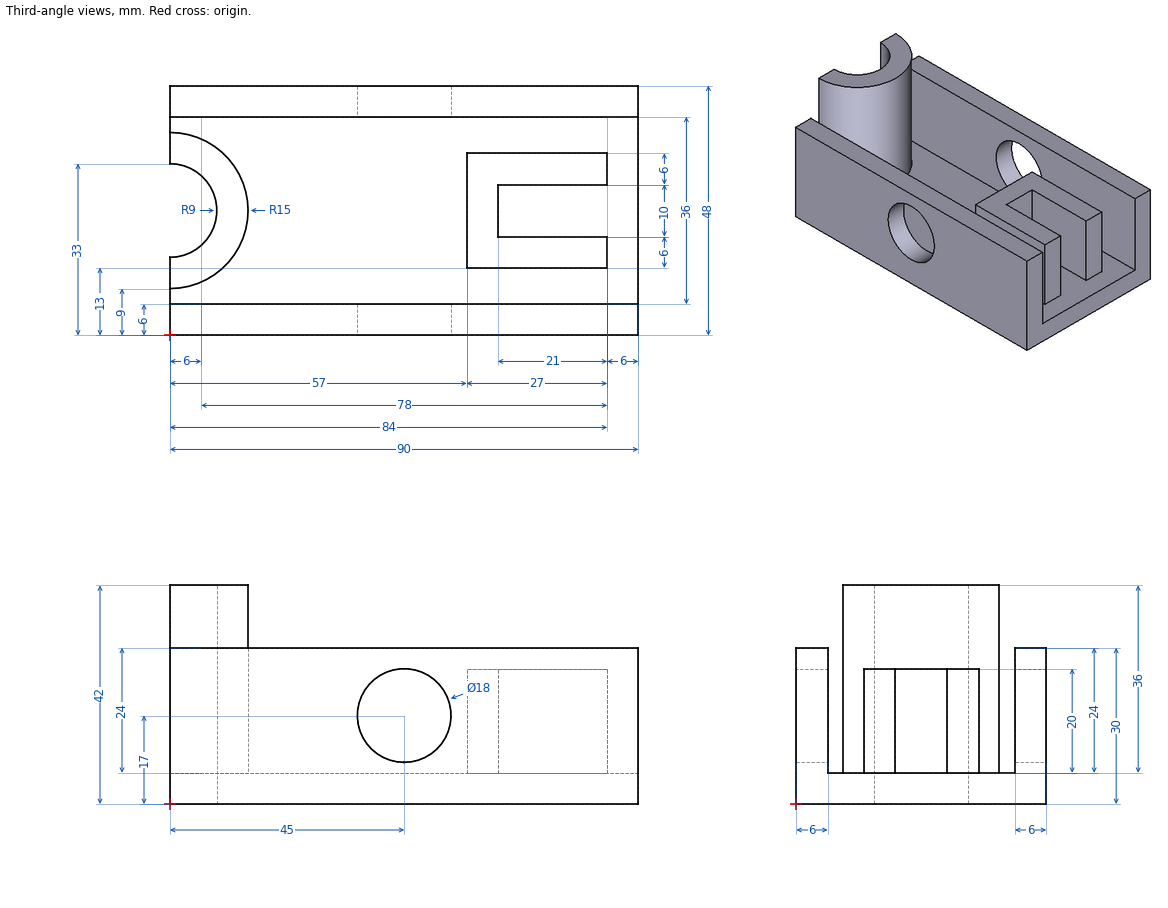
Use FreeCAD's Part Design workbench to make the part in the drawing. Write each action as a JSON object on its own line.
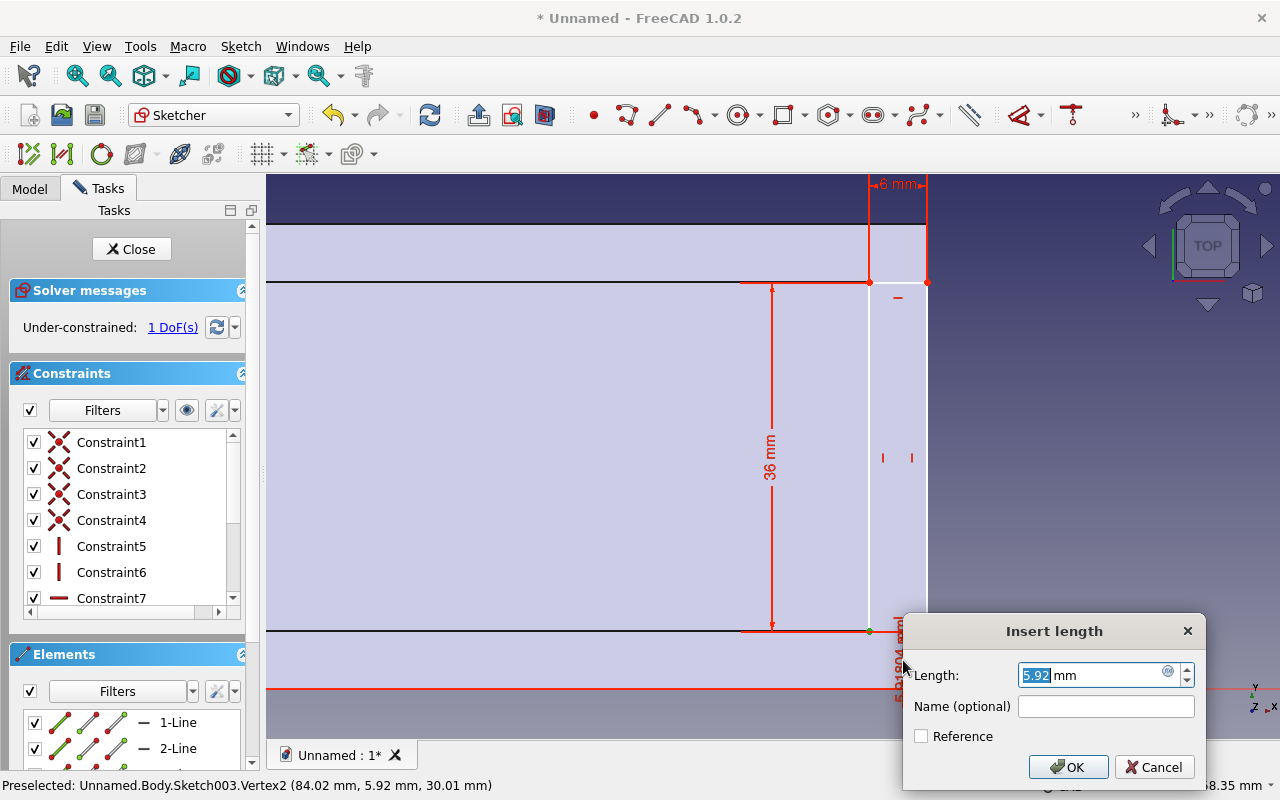
{"action": "type", "text": "6"}
{"action": "key", "text": "Return"}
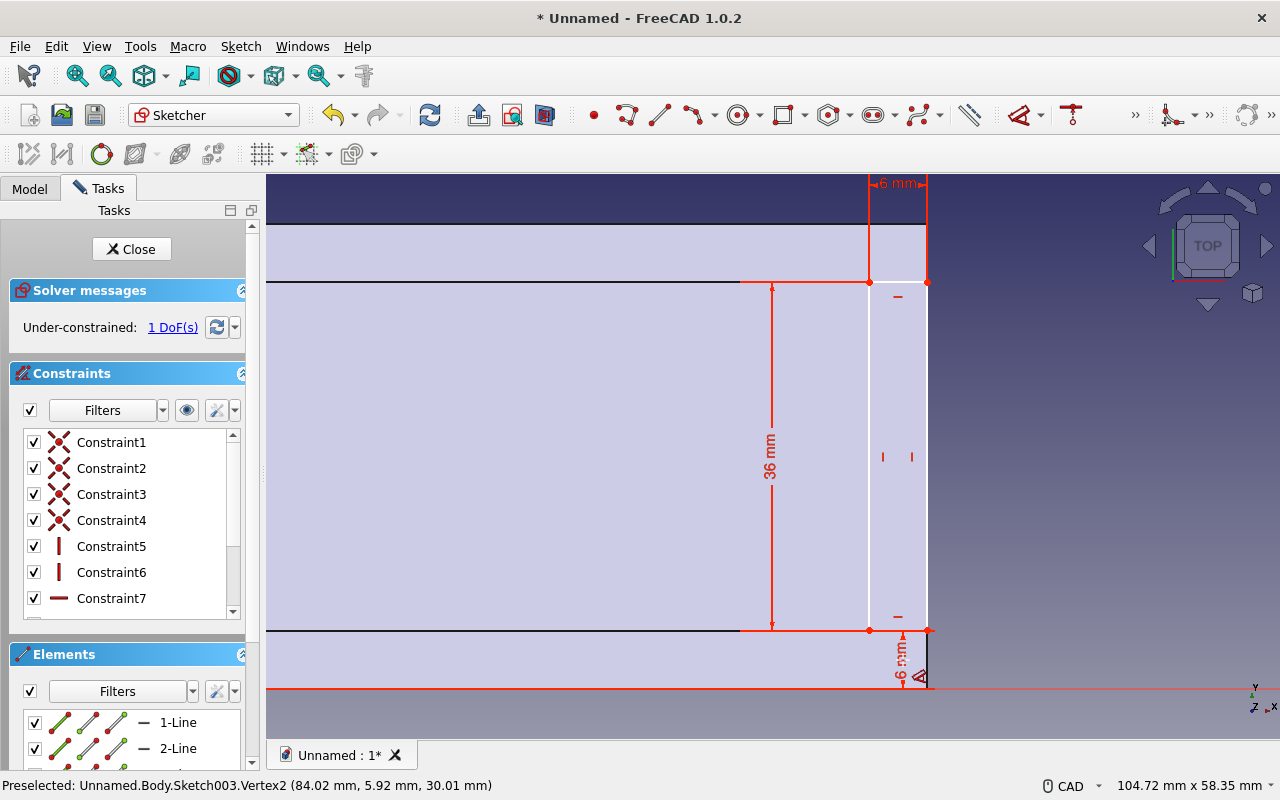
{"action": "left_click", "coordinate": [869, 282]}
{"action": "left_click", "coordinate": [581, 248]}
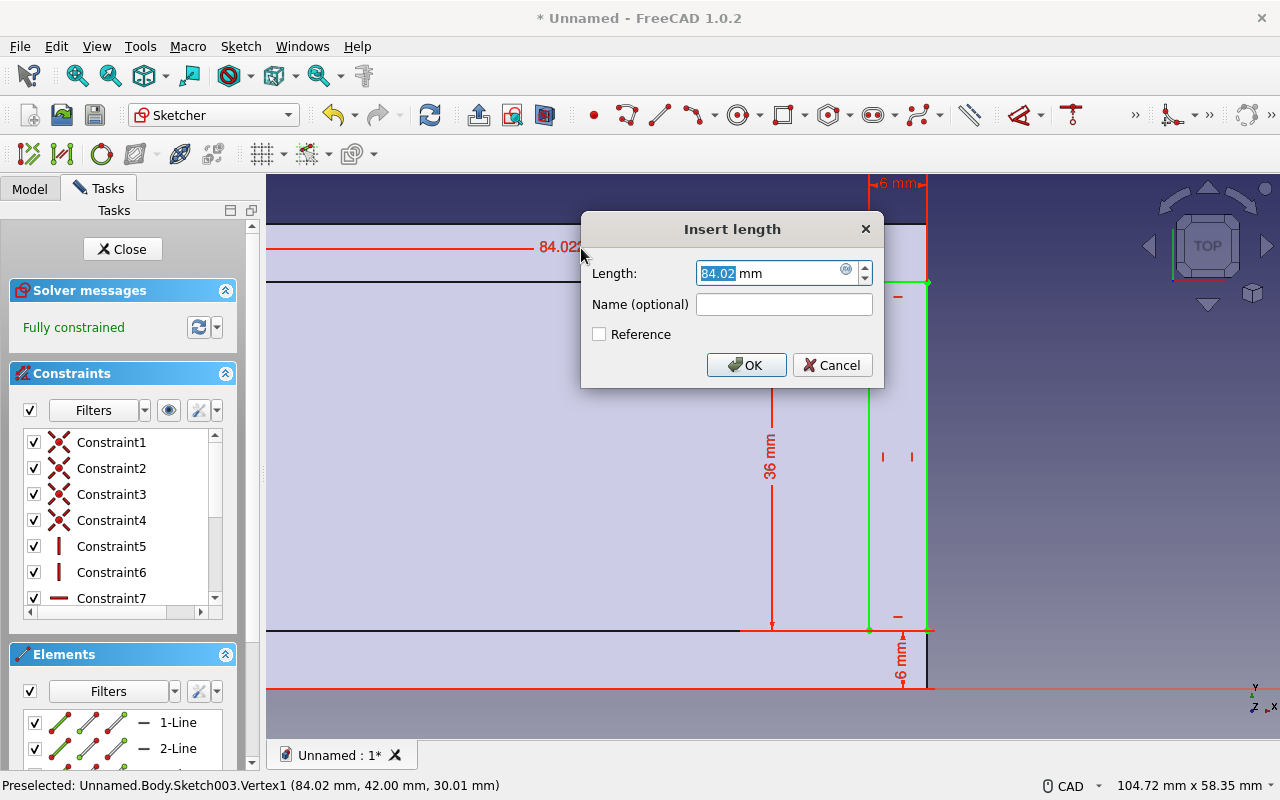
{"action": "type", "text": "84"}
{"action": "key", "text": "Return"}
{"action": "key", "text": "Escape"}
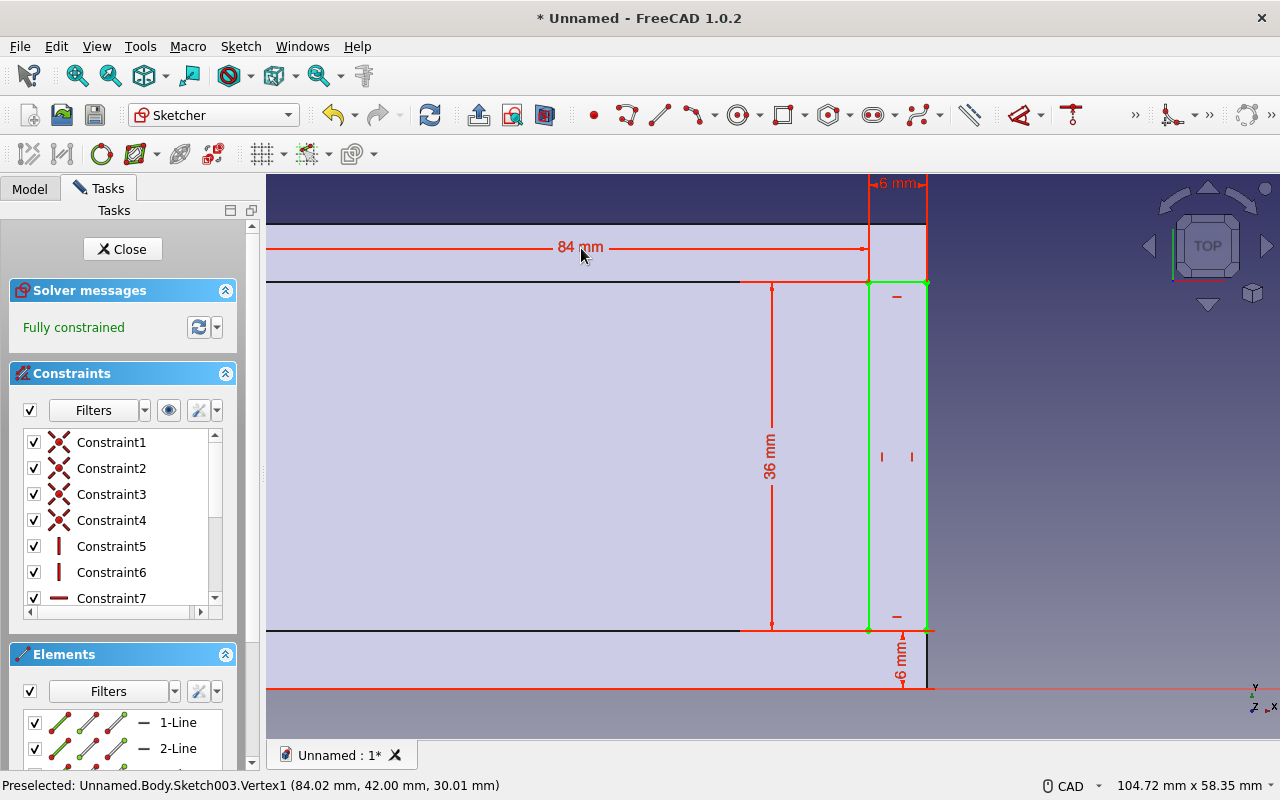
{"action": "left_click", "coordinate": [123, 249]}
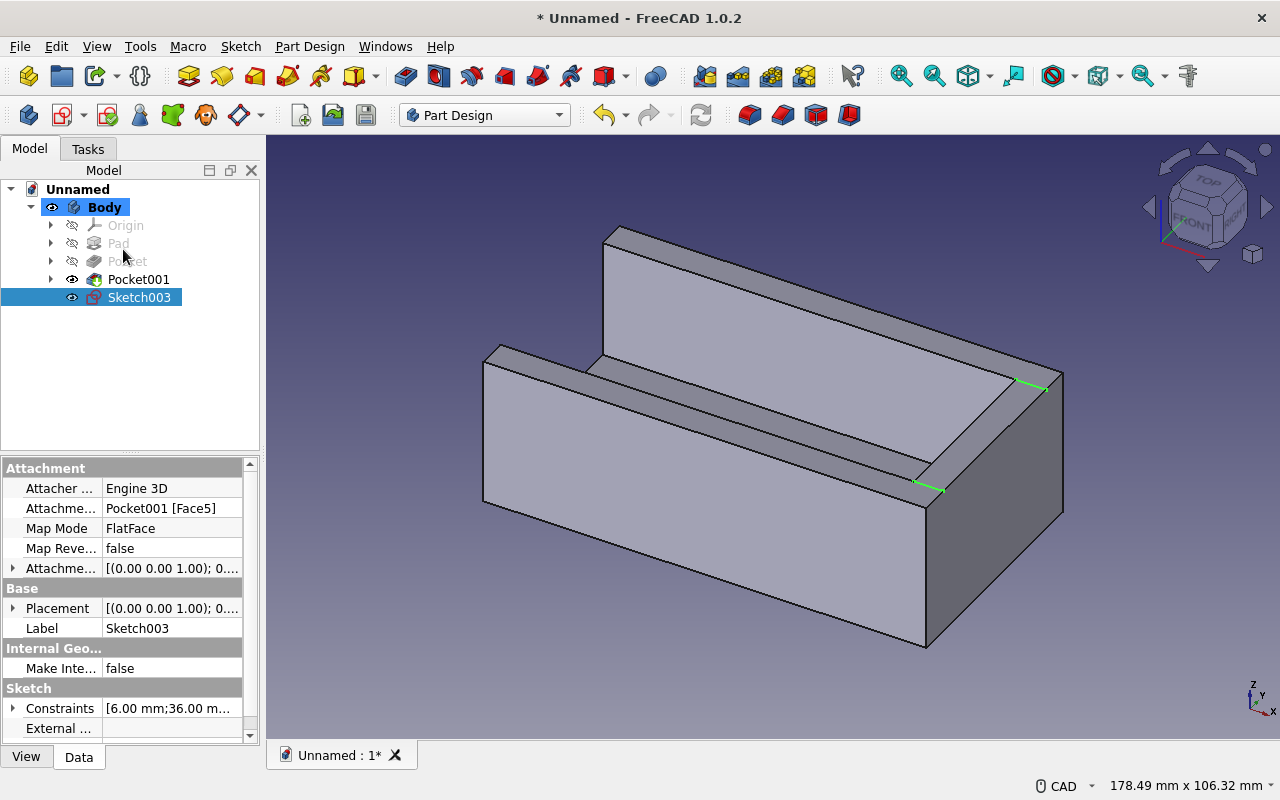
{"action": "left_click", "coordinate": [406, 76]}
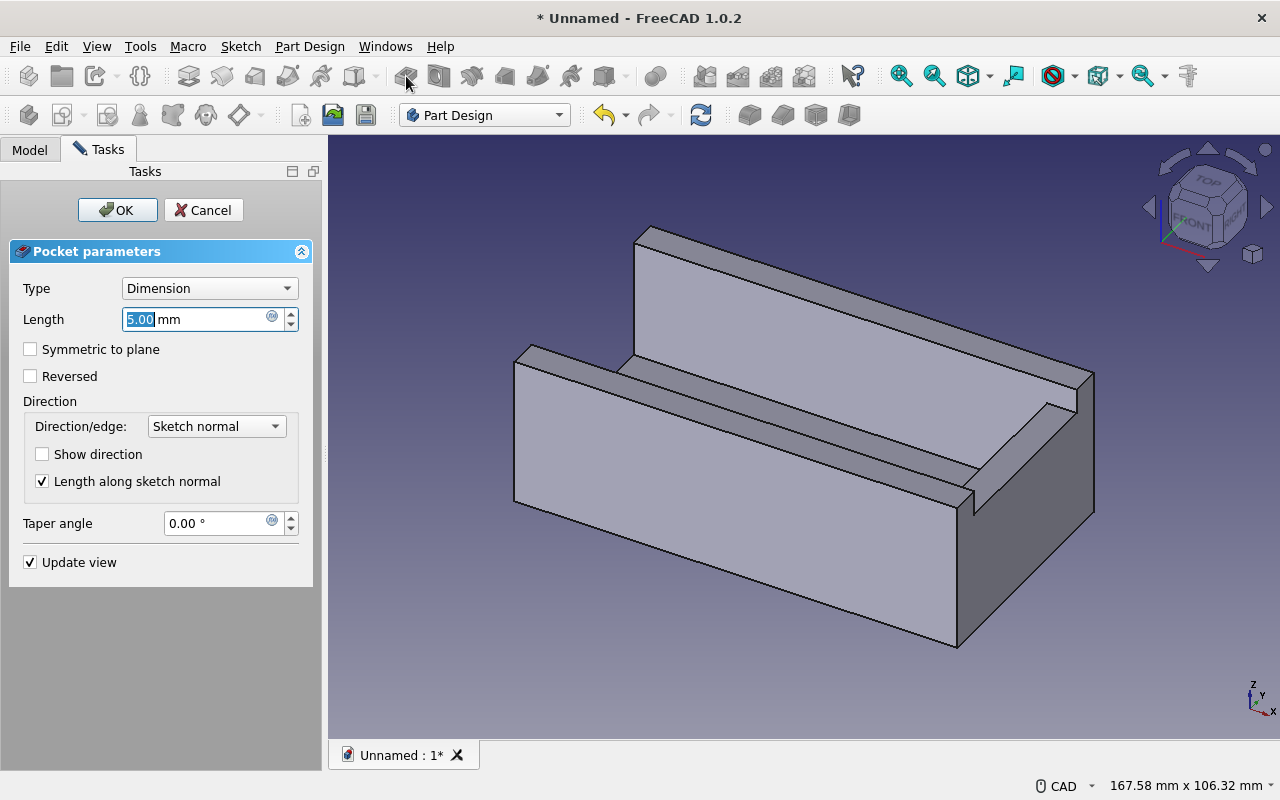
{"action": "type", "text": "24"}
{"action": "key", "text": "Tab"}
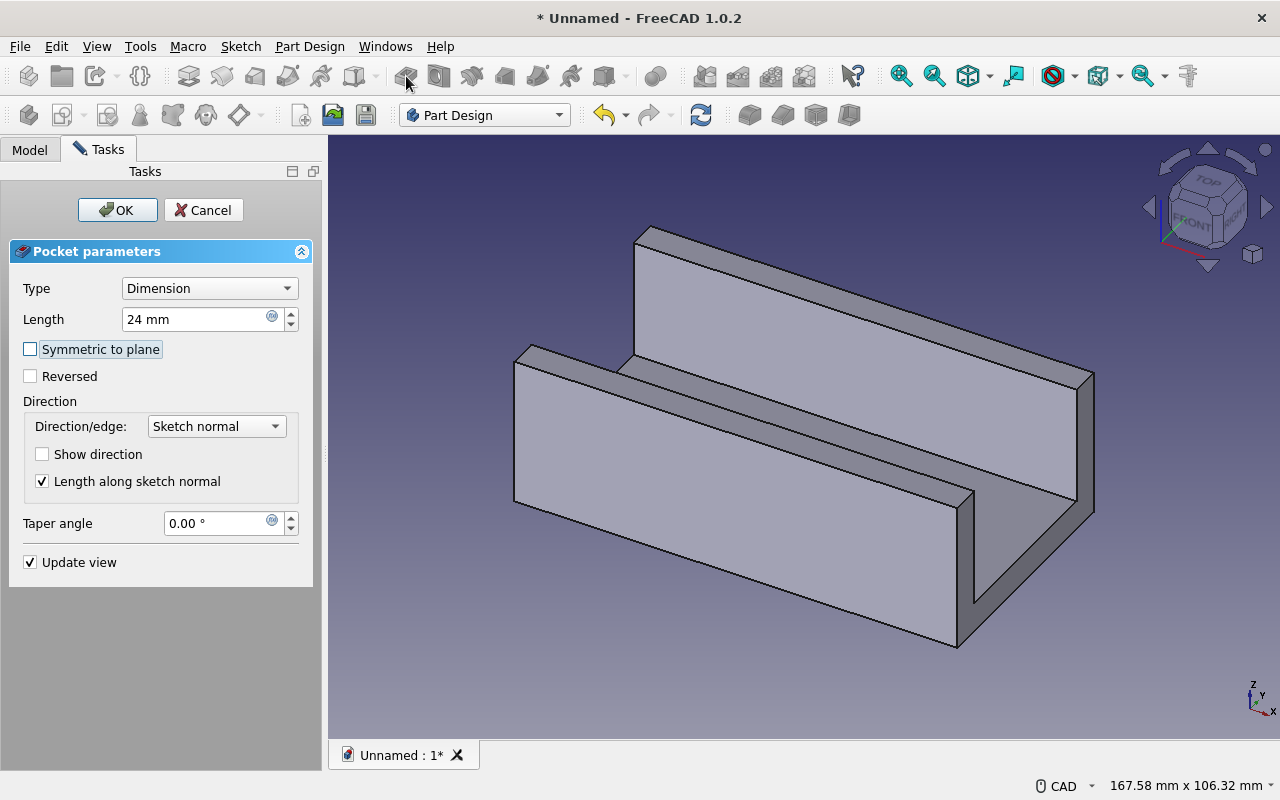
{"action": "left_click", "coordinate": [118, 210]}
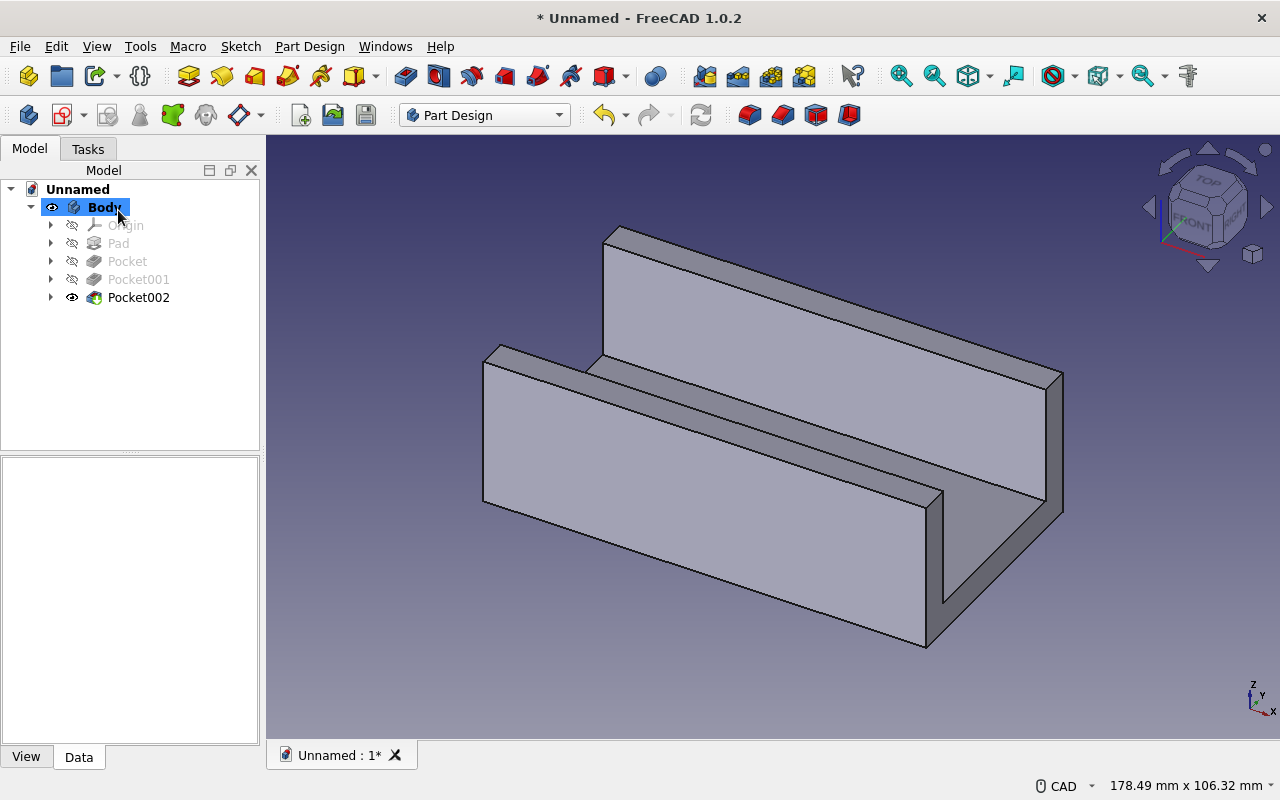
{"action": "key", "text": "0"}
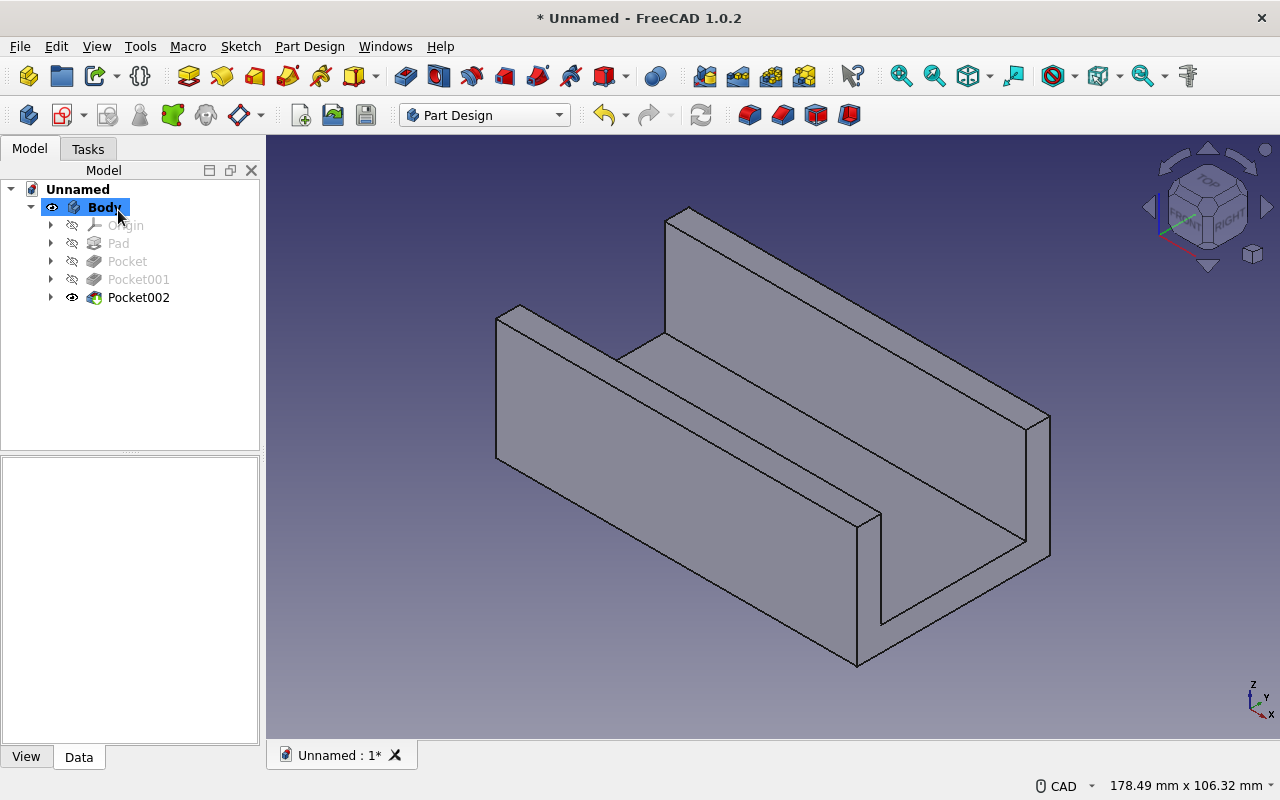
{"action": "left_click", "coordinate": [897, 525]}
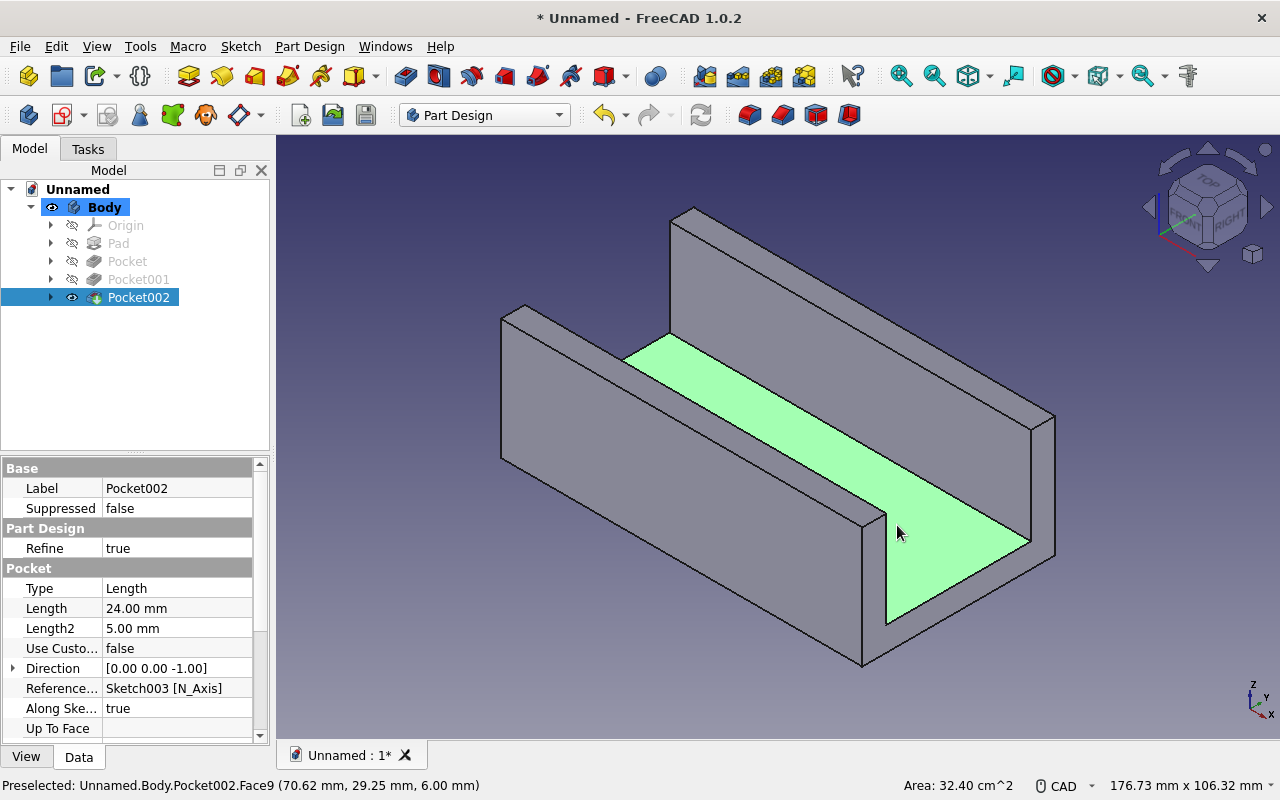
{"action": "left_click", "coordinate": [62, 116]}